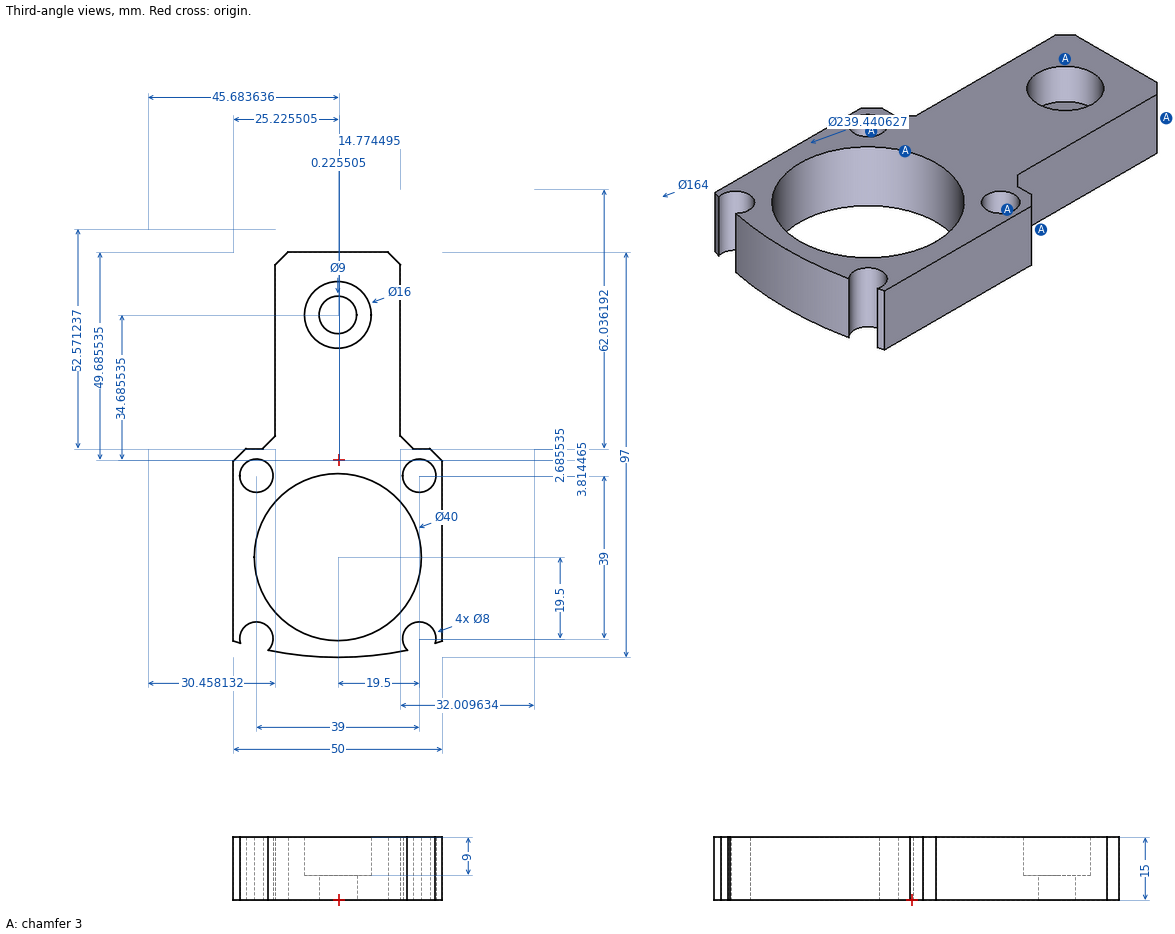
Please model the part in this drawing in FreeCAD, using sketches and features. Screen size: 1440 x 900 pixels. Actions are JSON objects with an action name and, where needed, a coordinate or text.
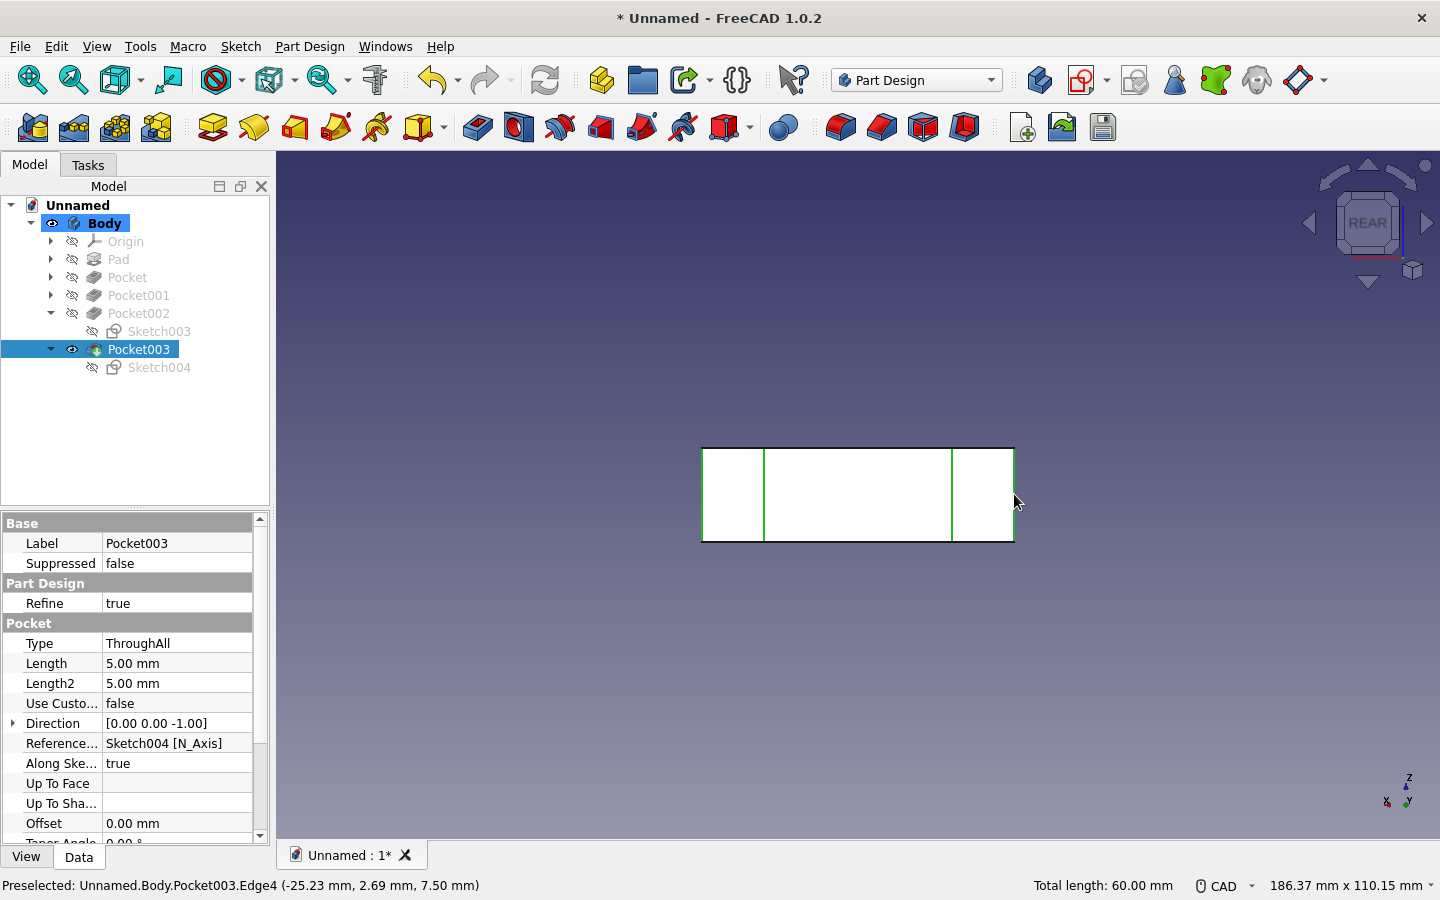
{"action": "key", "text": "6"}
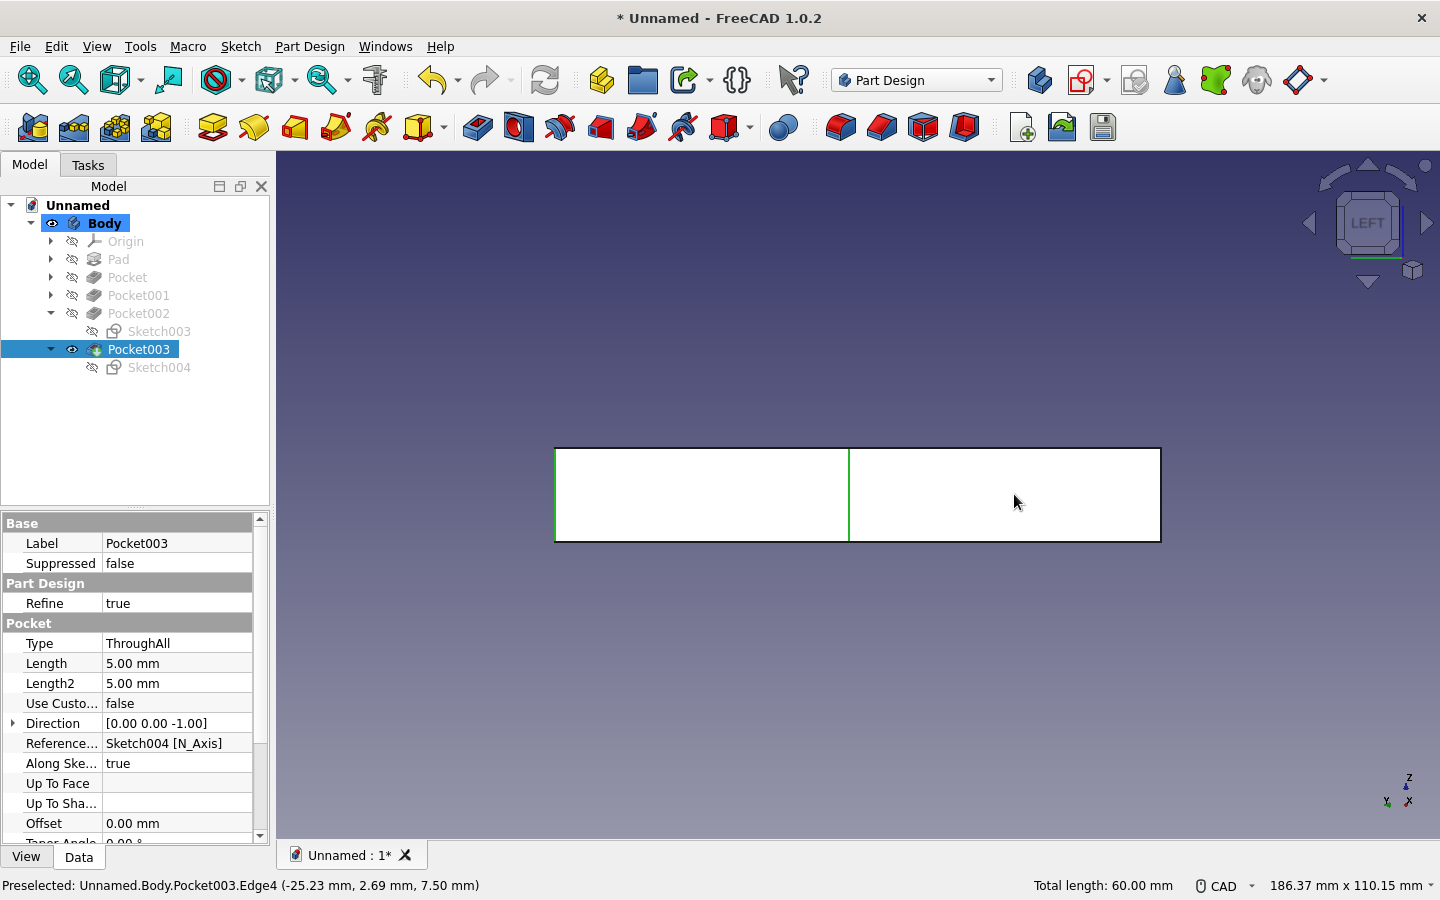
{"action": "key", "text": "v 3"}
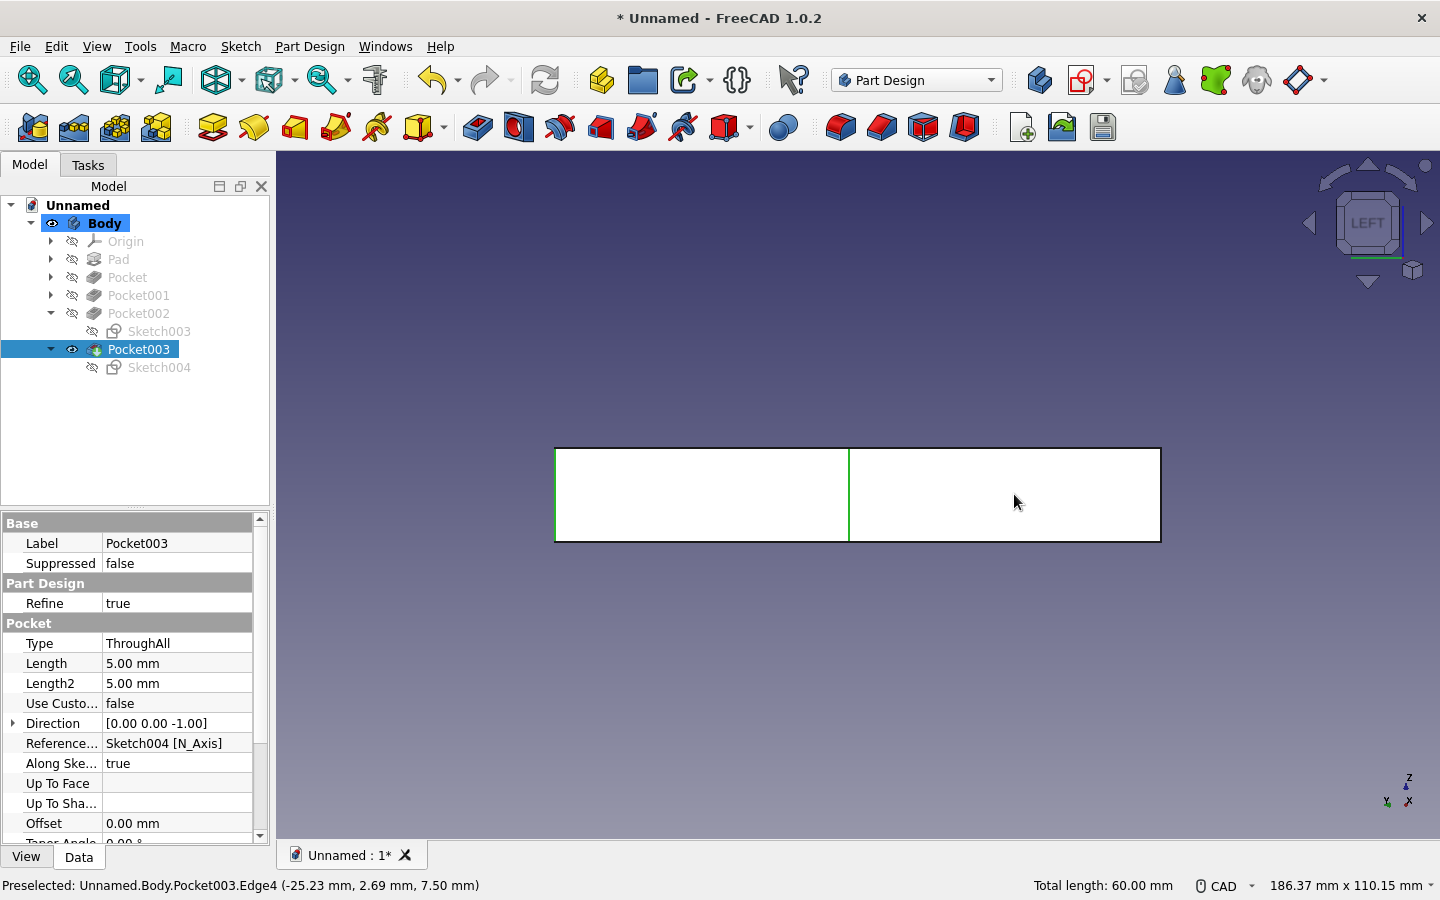
{"action": "key", "text": "0"}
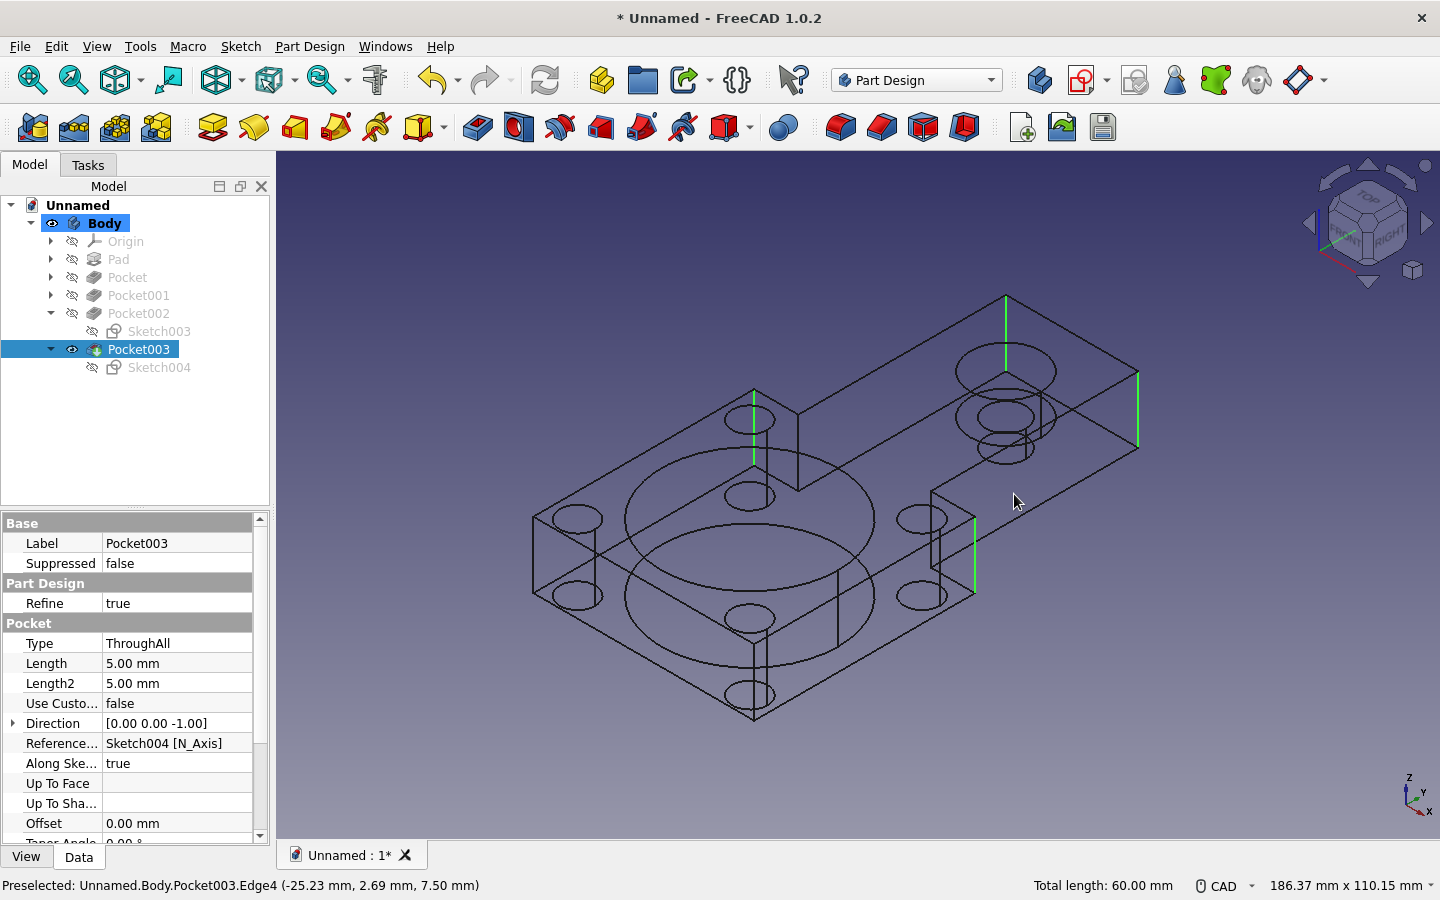
{"action": "left_click", "coordinate": [931, 521], "text": "ctrl"}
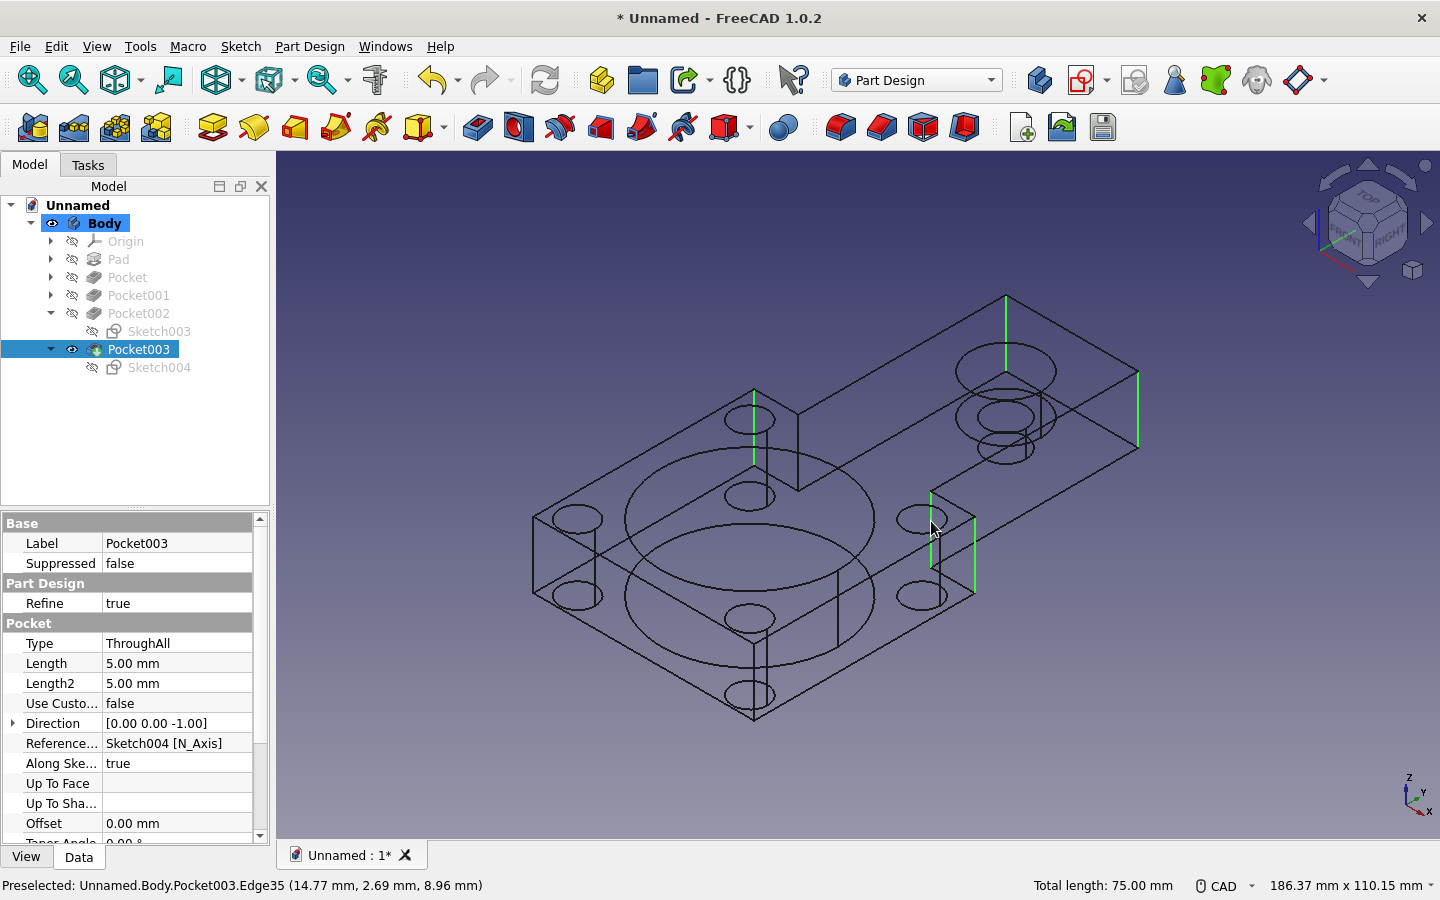
{"action": "left_click", "coordinate": [798, 444], "text": "ctrl"}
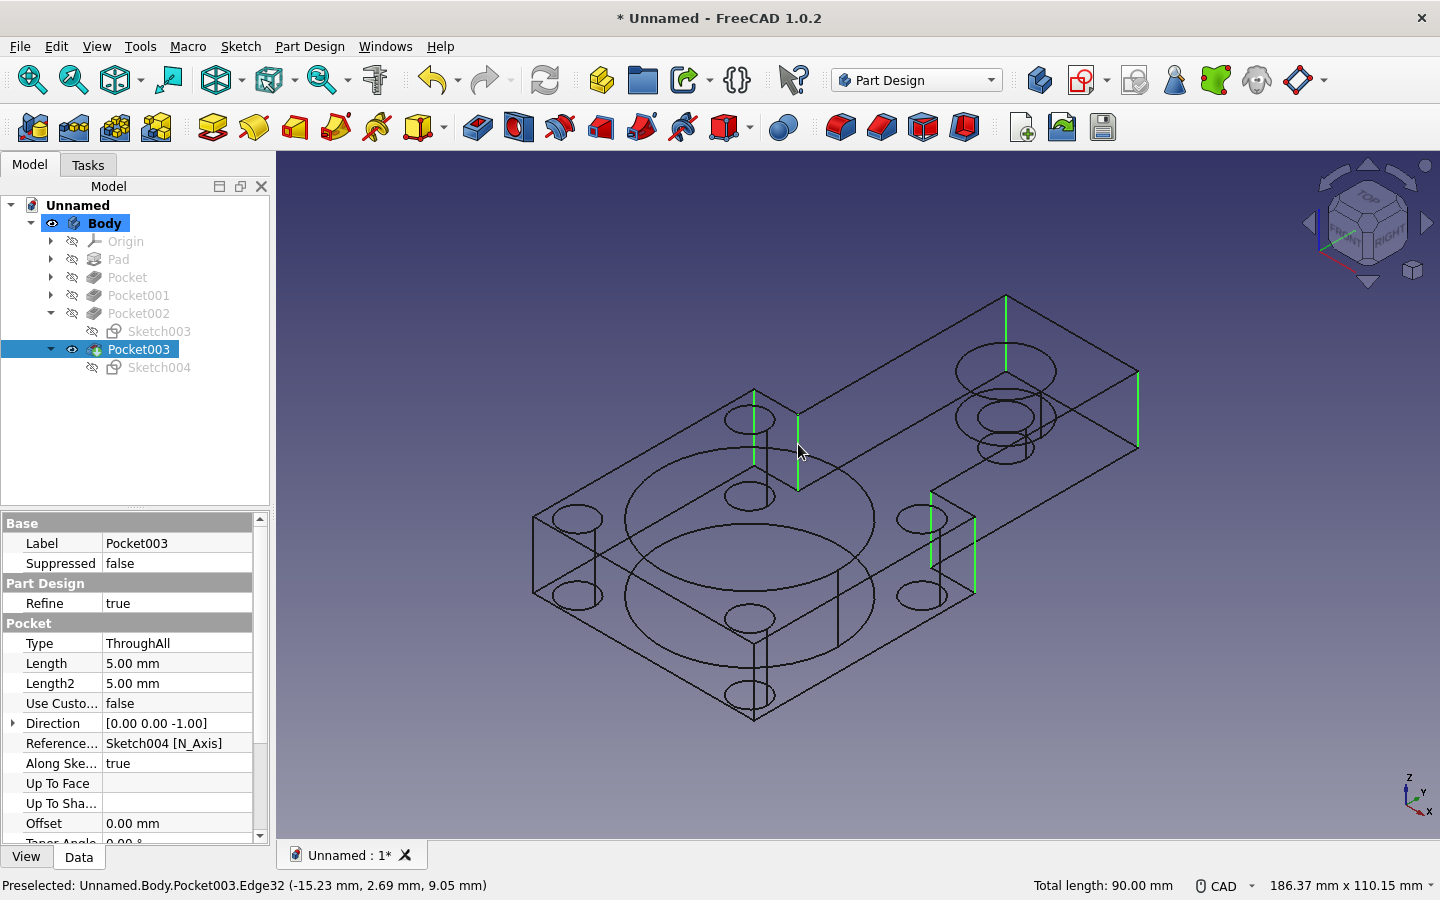
{"action": "key", "text": "v 1"}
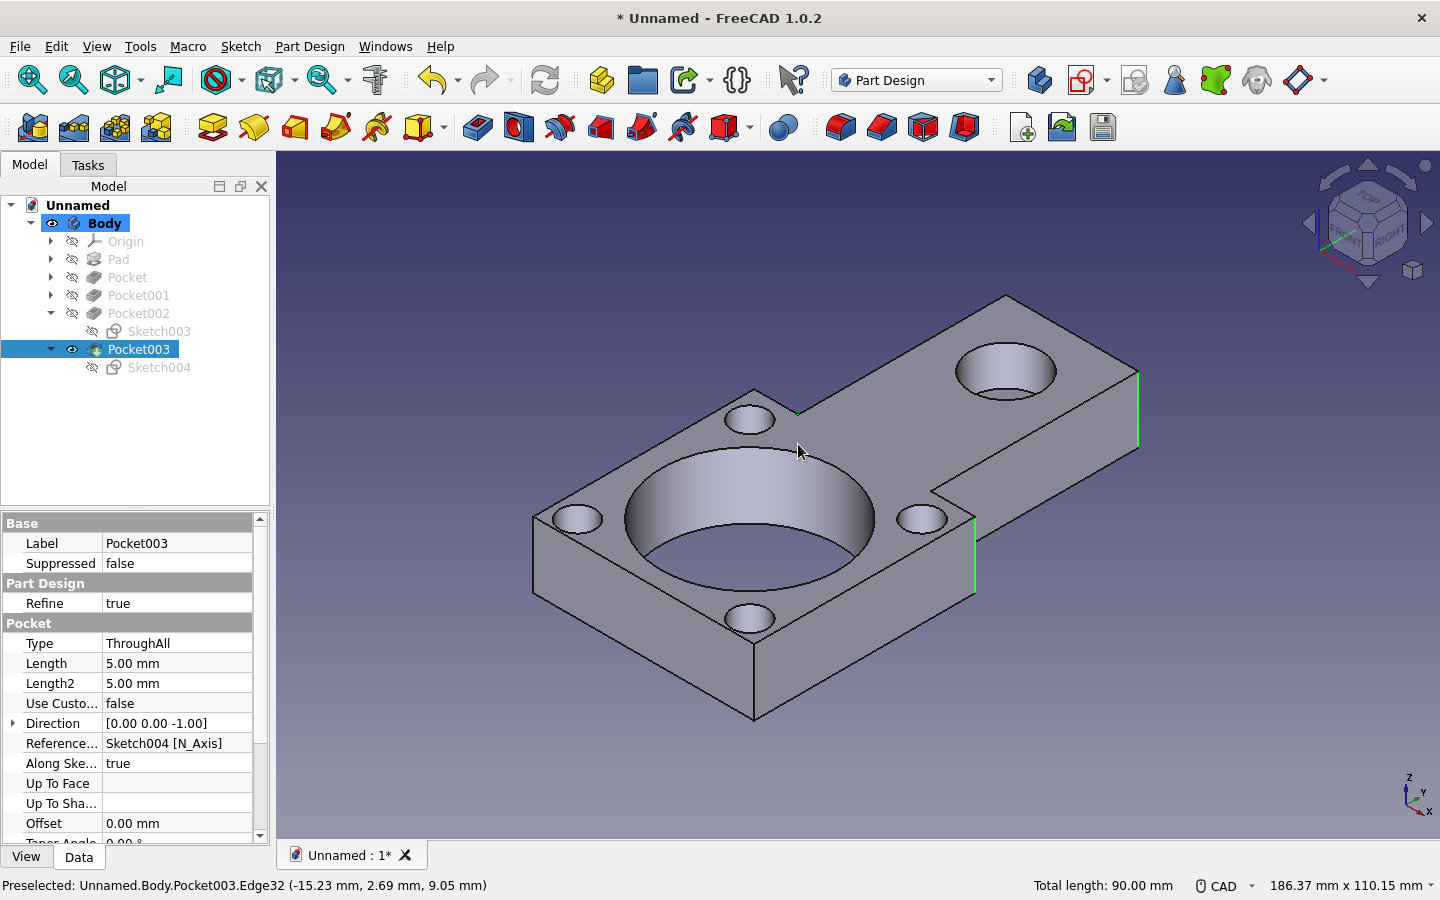
{"action": "left_click", "coordinate": [882, 128]}